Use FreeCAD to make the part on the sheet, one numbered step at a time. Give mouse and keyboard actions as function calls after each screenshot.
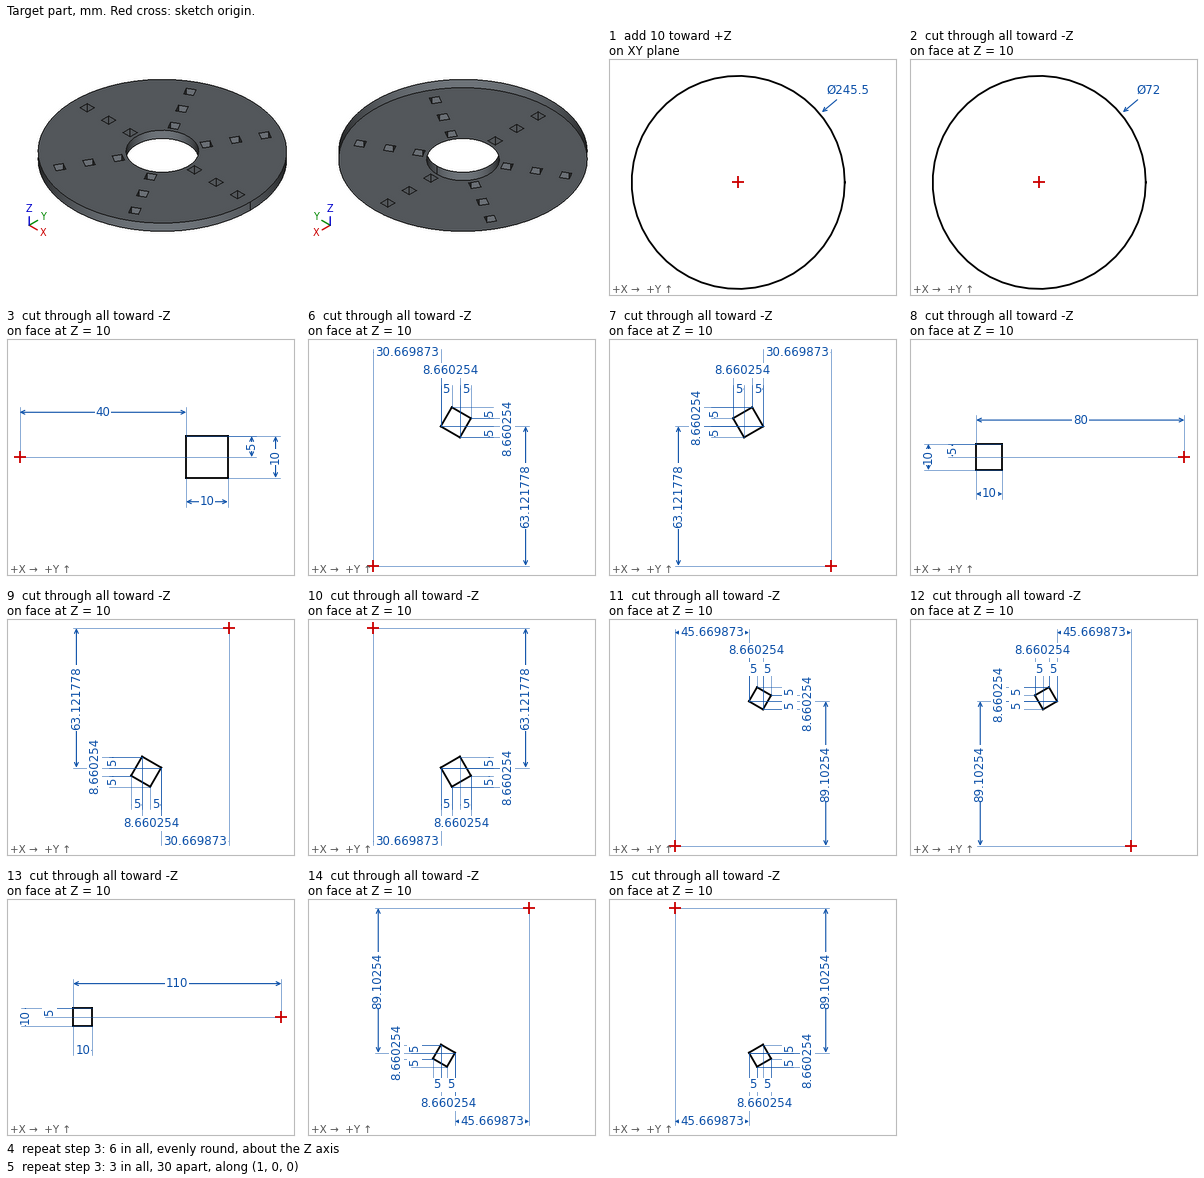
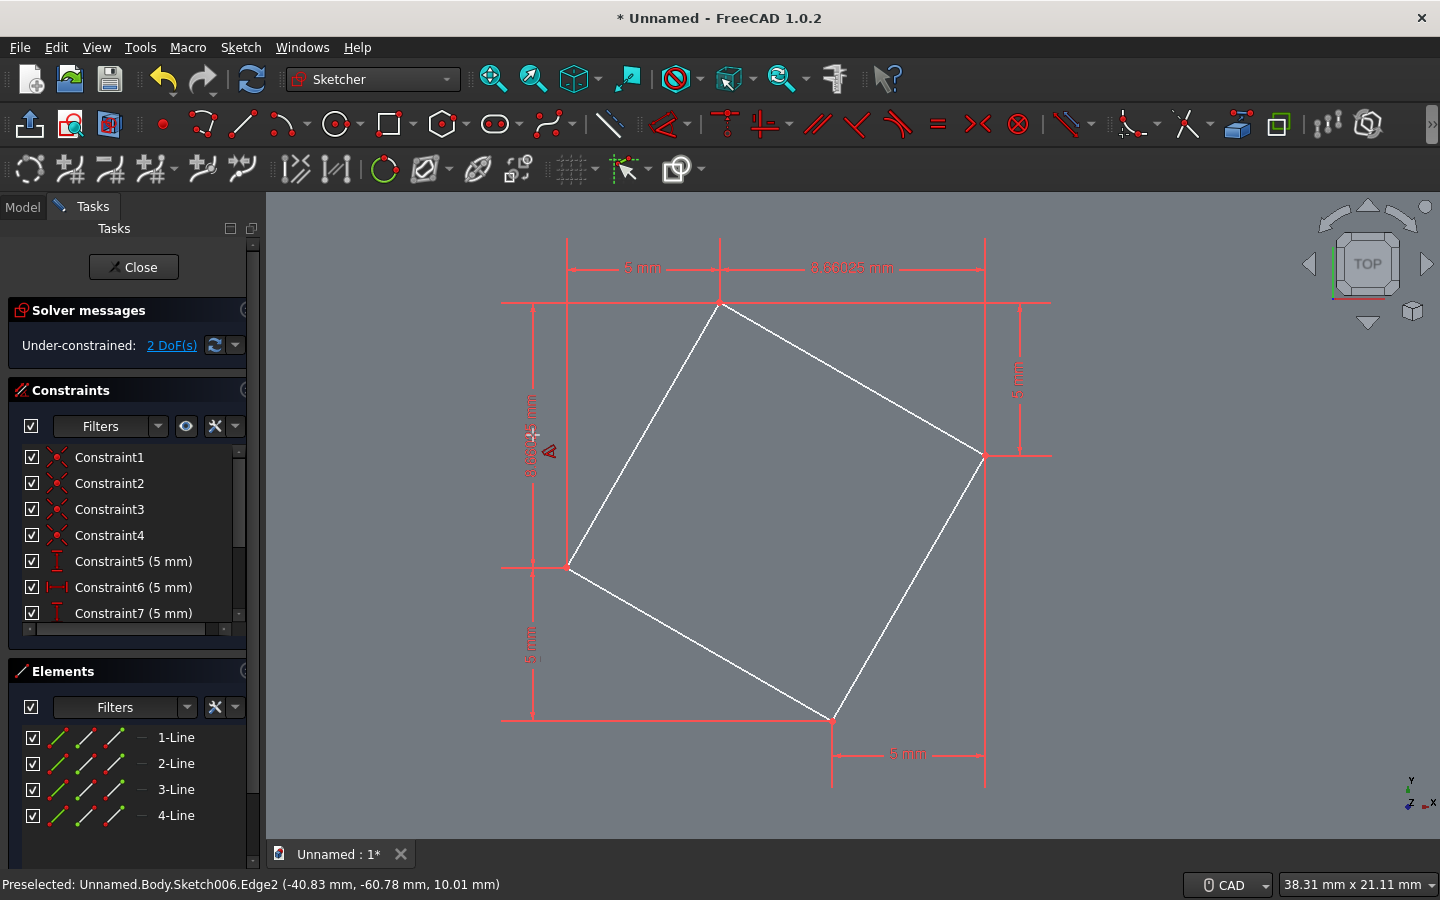
click(985, 456)
click(1130, 490)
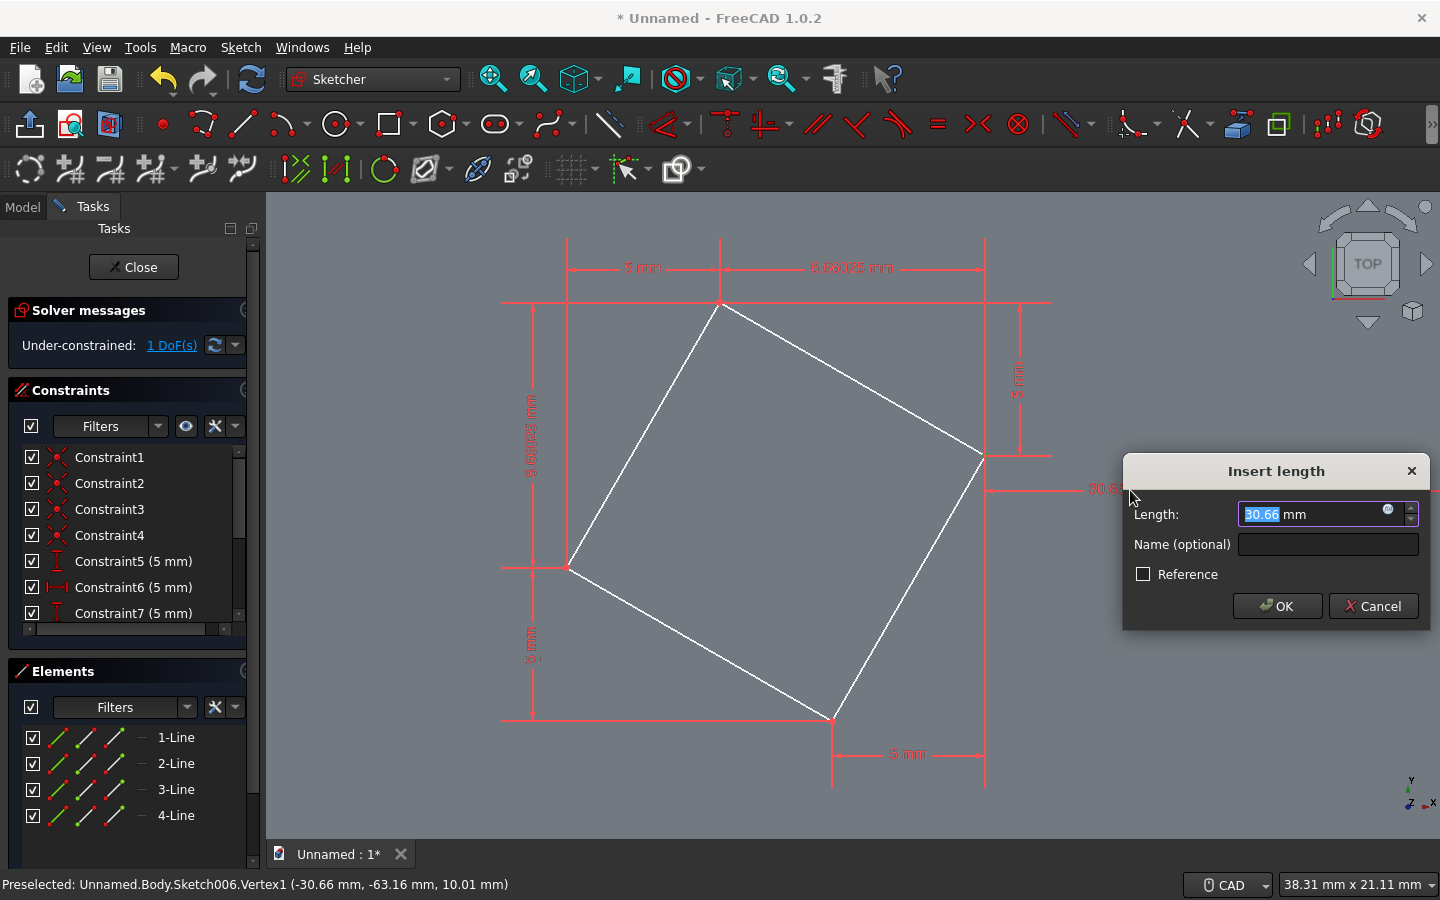
text(30.669873)
key(Return)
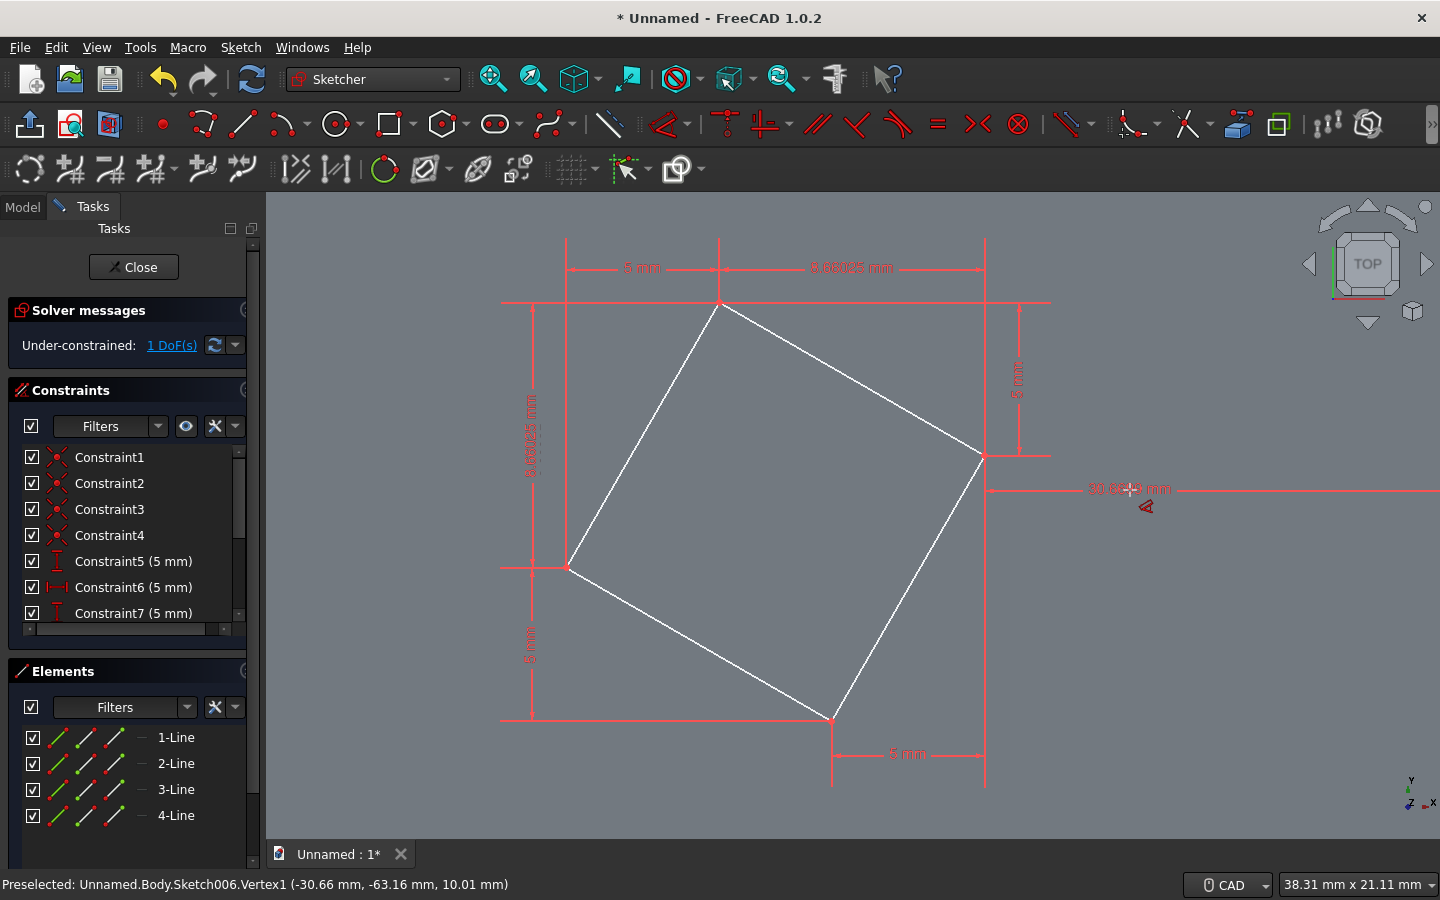
click(985, 456)
click(951, 338)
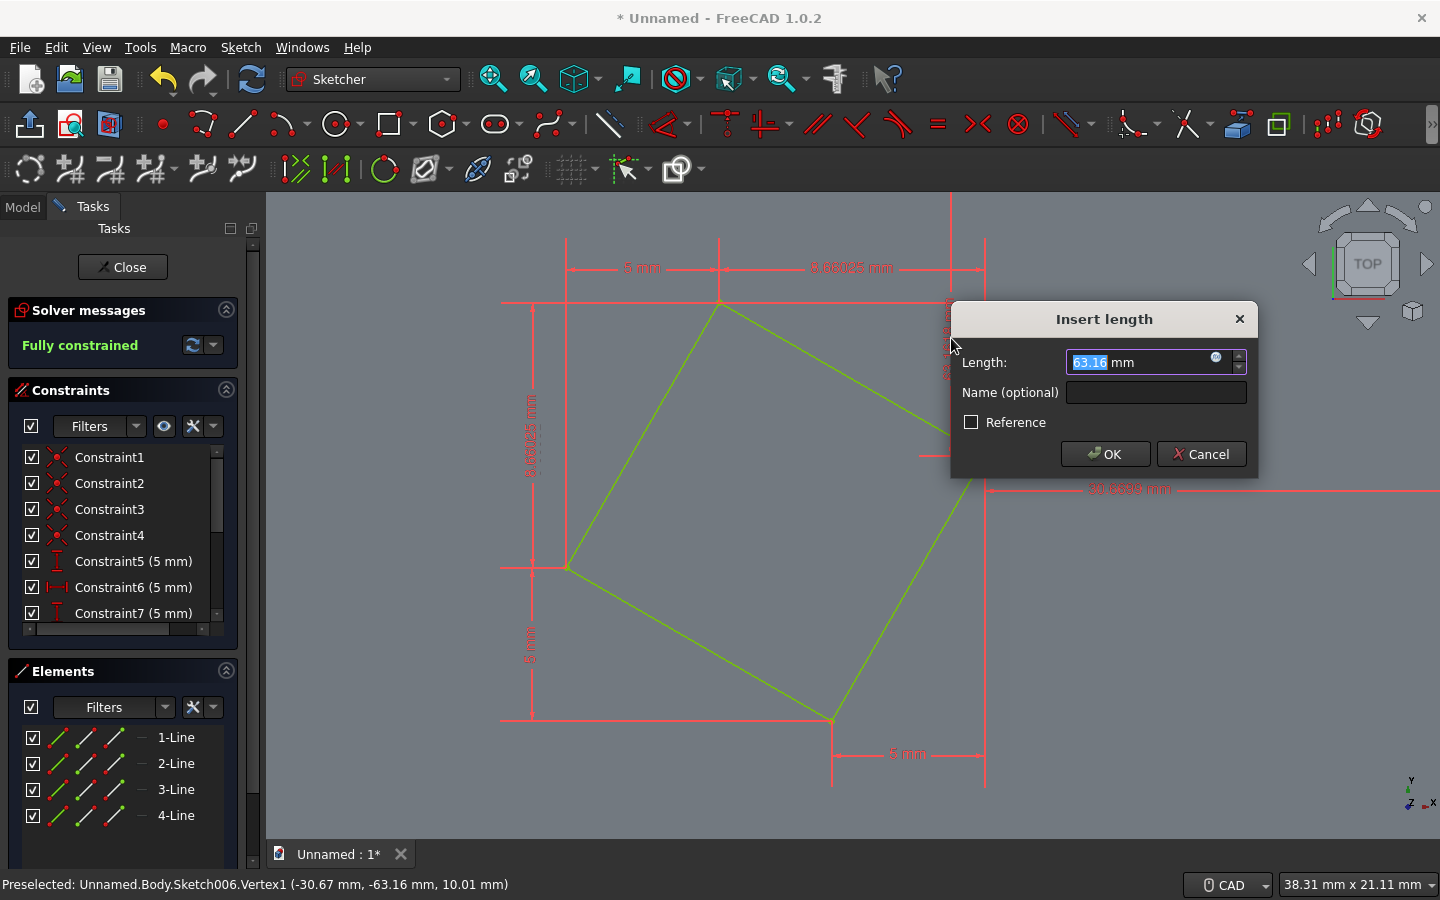
text(63.121778)
key(Return)
key(Escape)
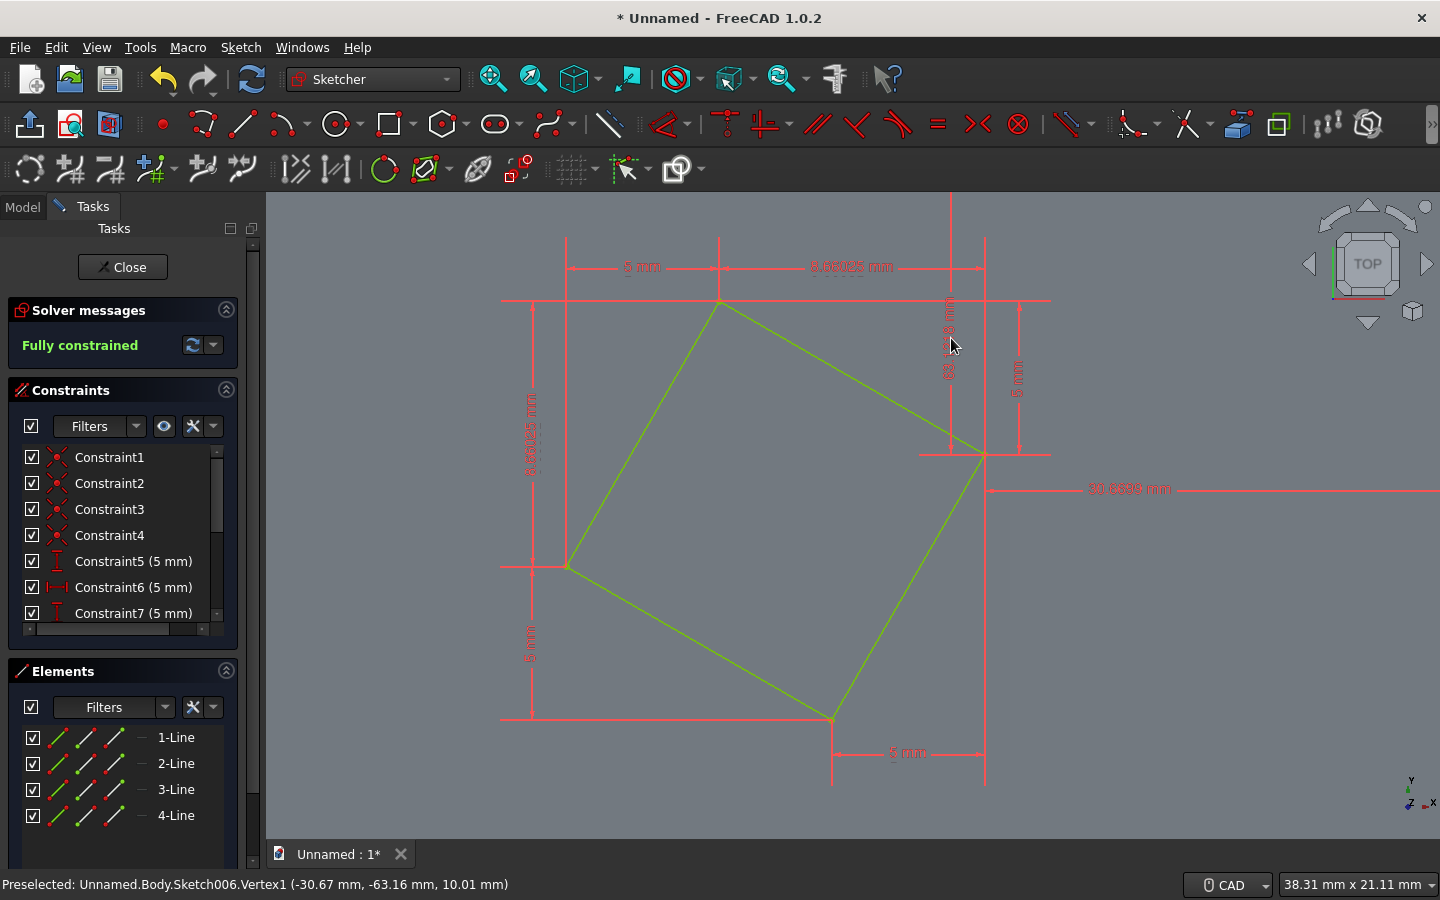
click(123, 267)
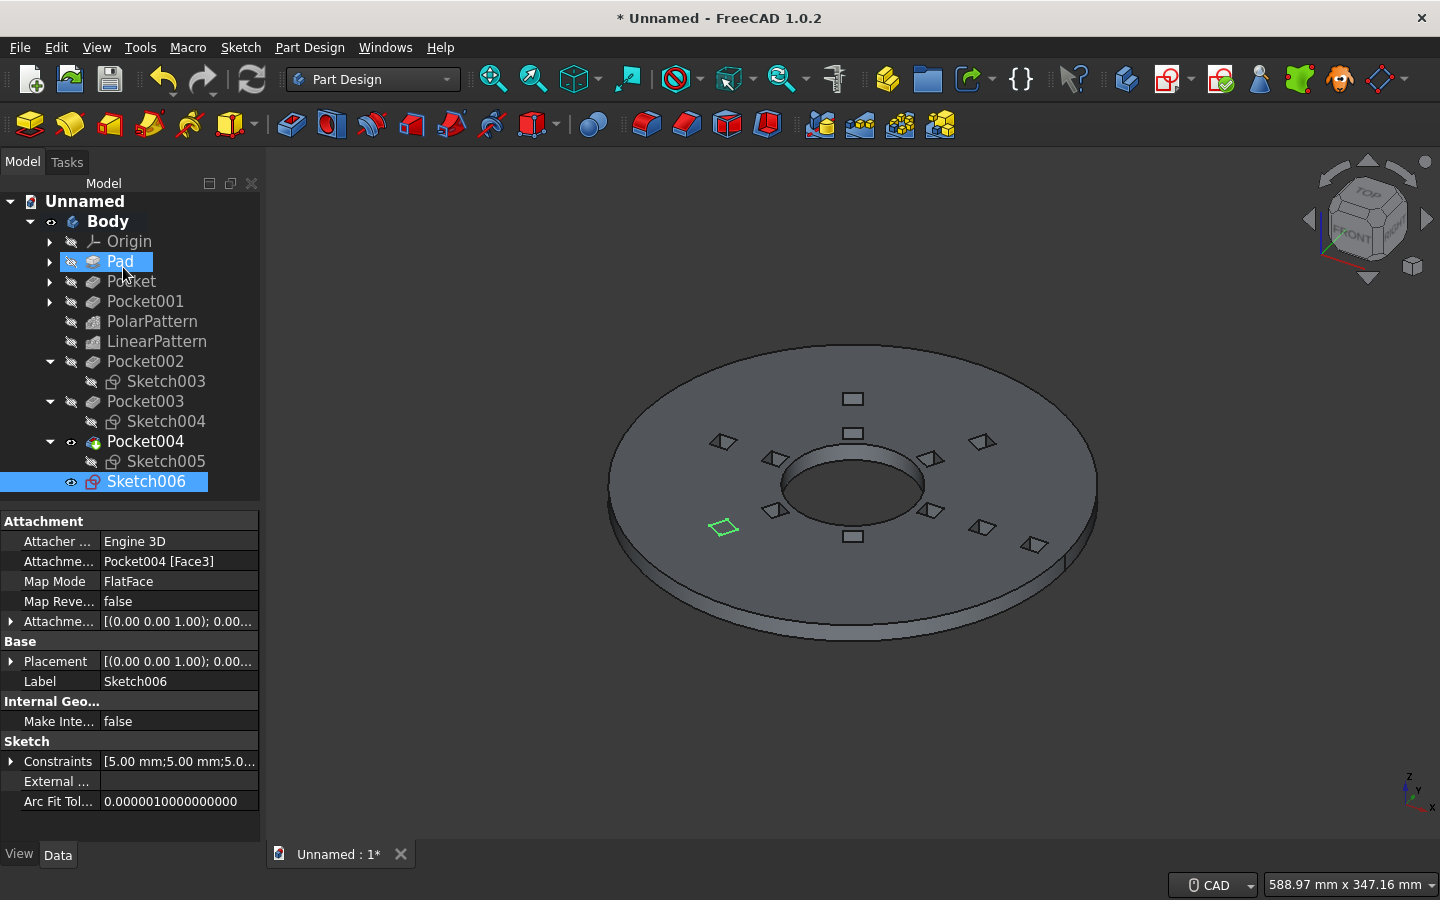
click(292, 124)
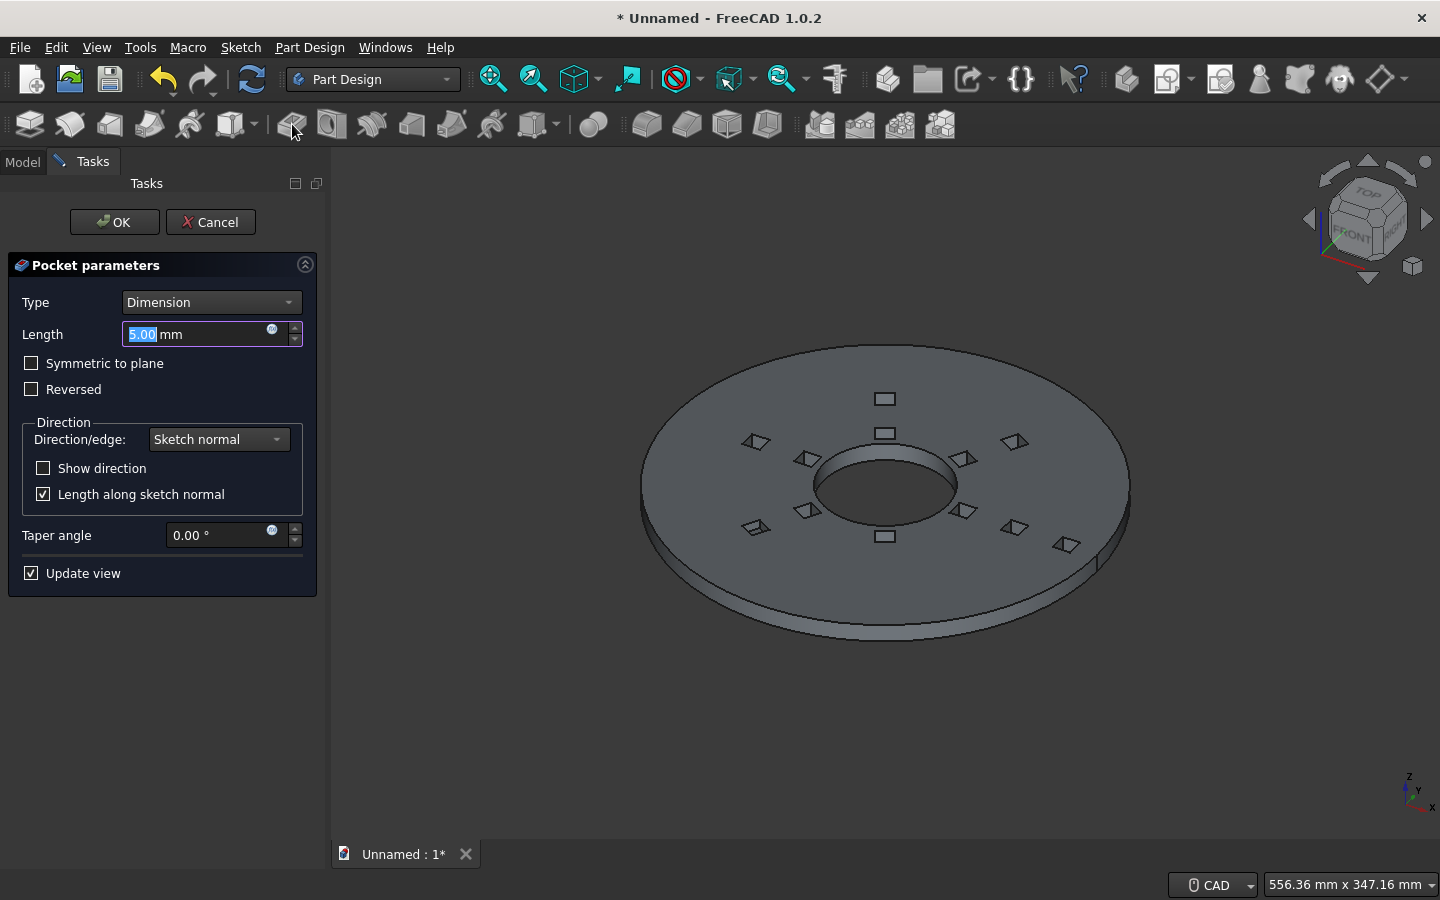
click(212, 302)